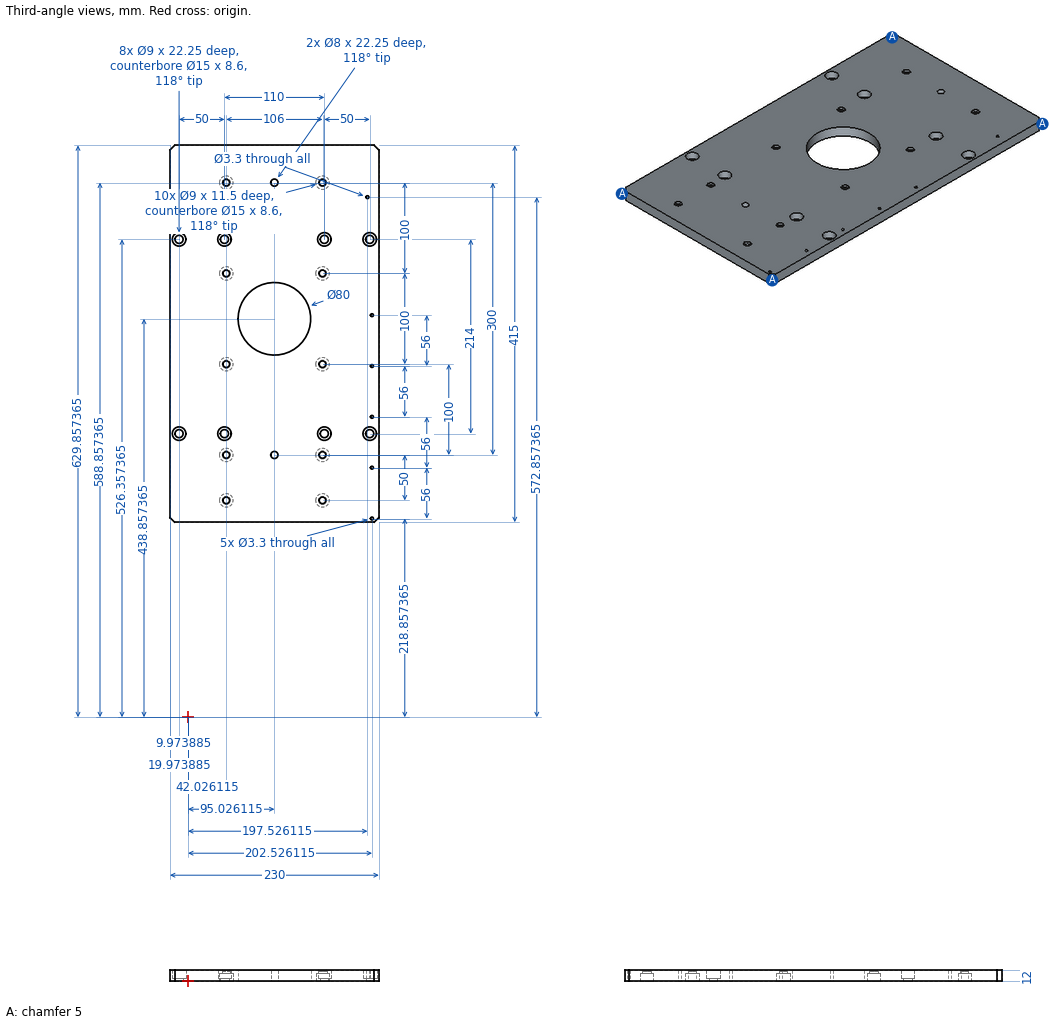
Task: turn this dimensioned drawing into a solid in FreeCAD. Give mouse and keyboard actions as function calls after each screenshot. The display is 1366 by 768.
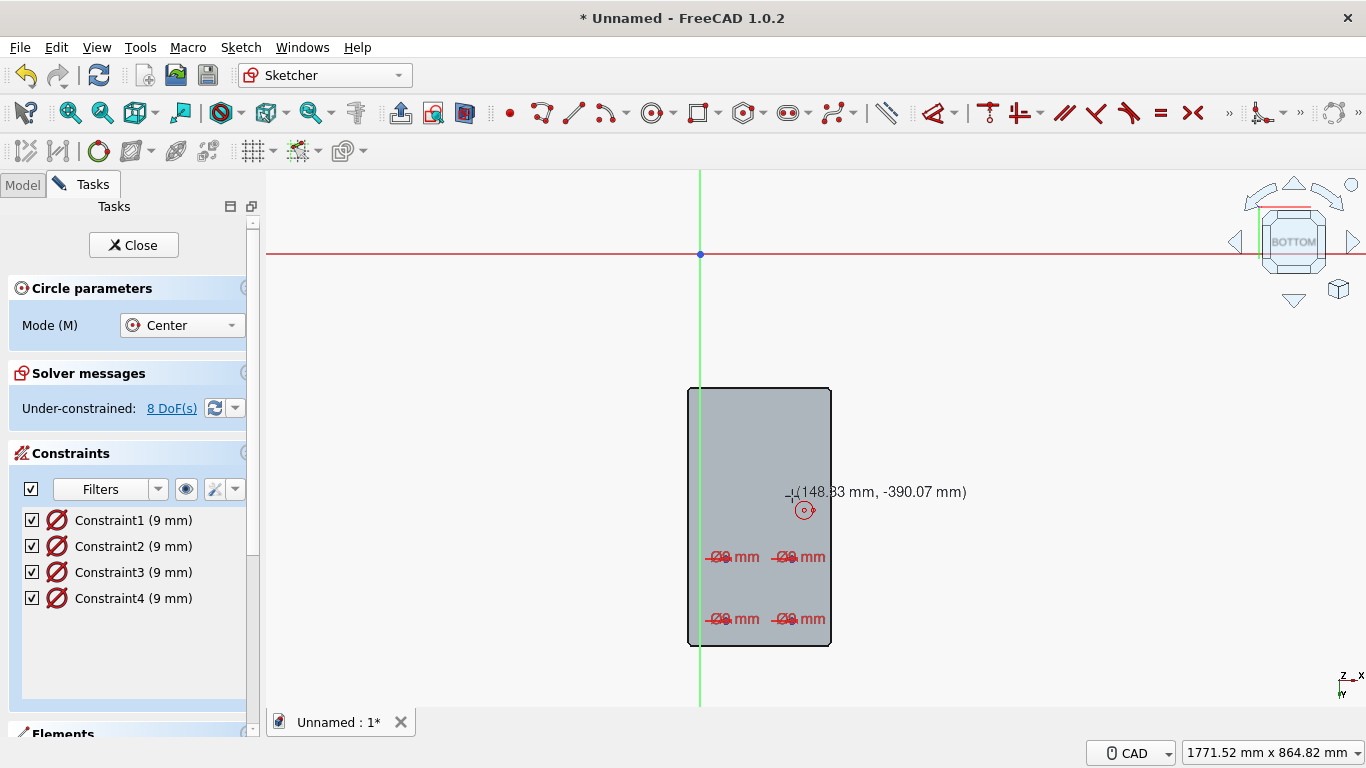
click(792, 496)
move(794, 494)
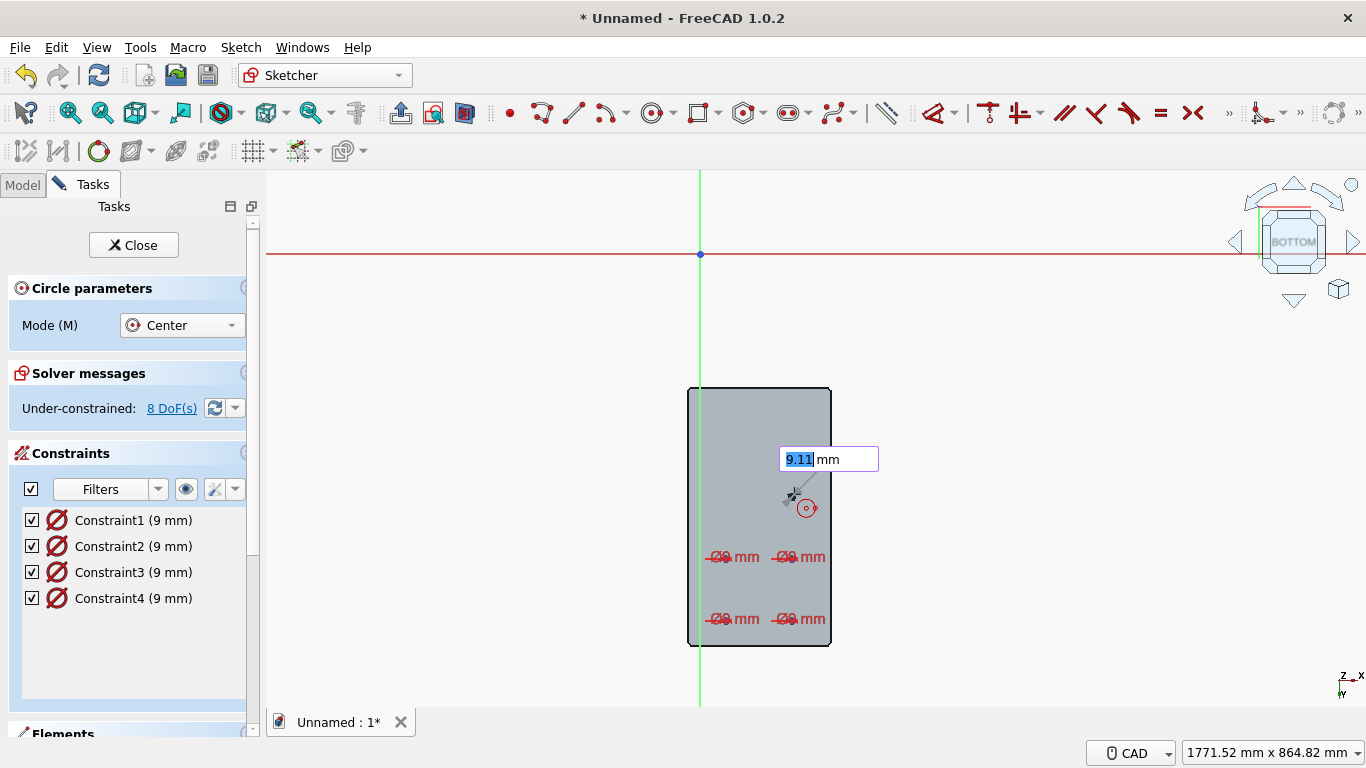
text(9)
key(Return)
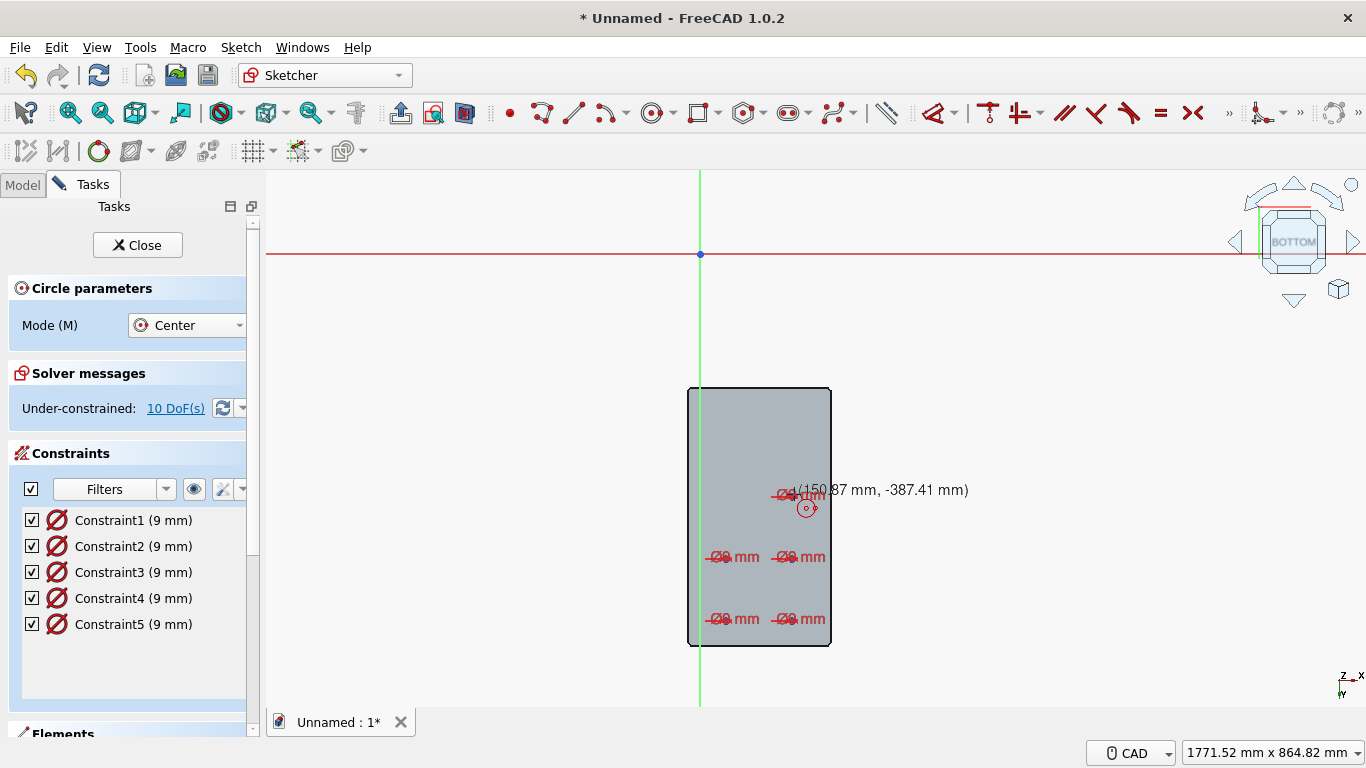
scroll(726, 496, up, 11)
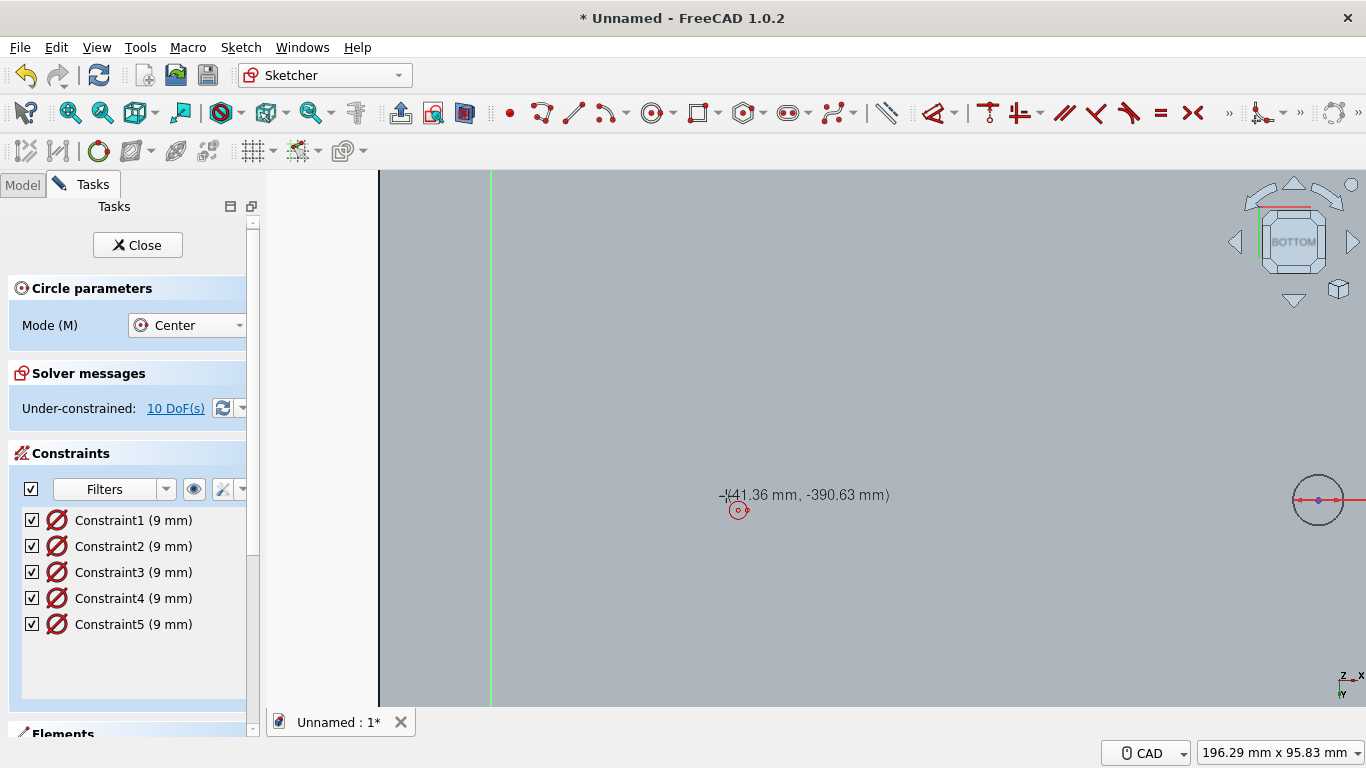
scroll(726, 496, down, 11)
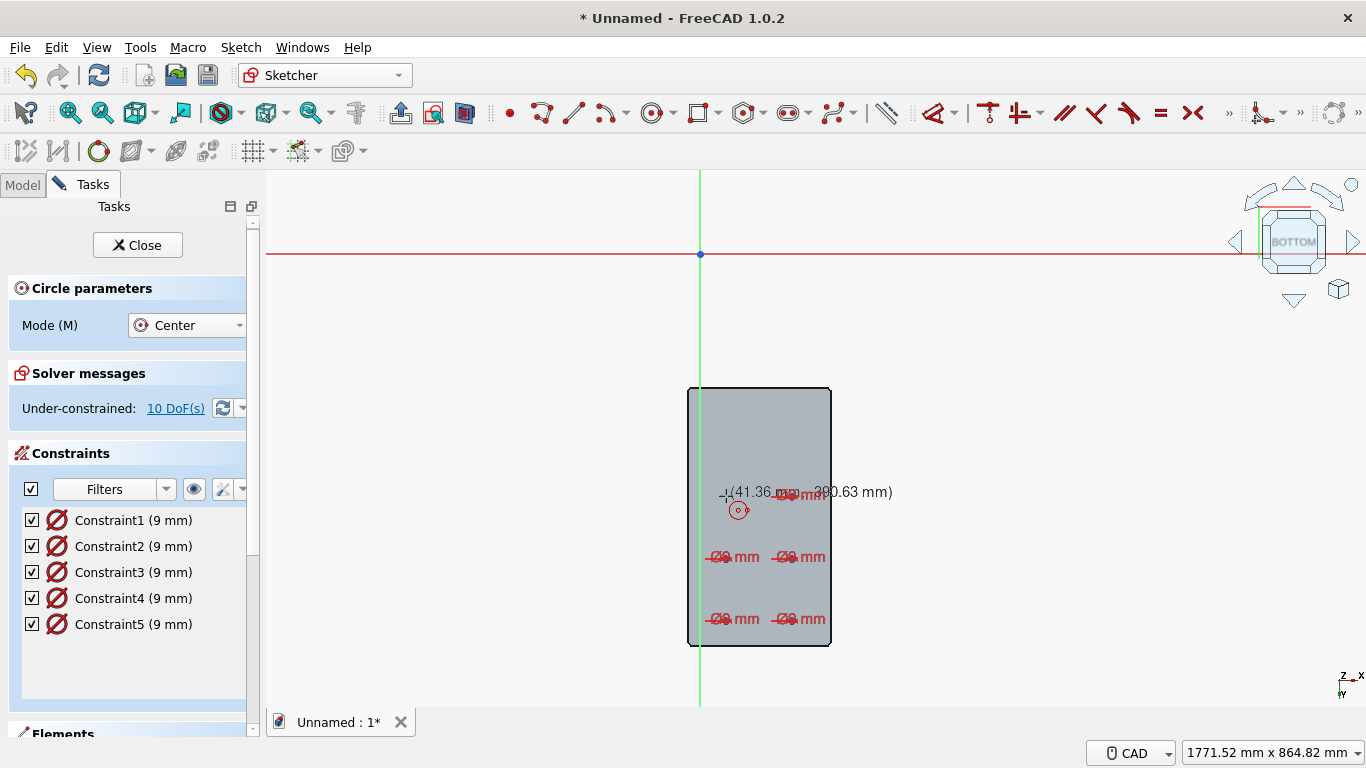
click(726, 496)
move(728, 494)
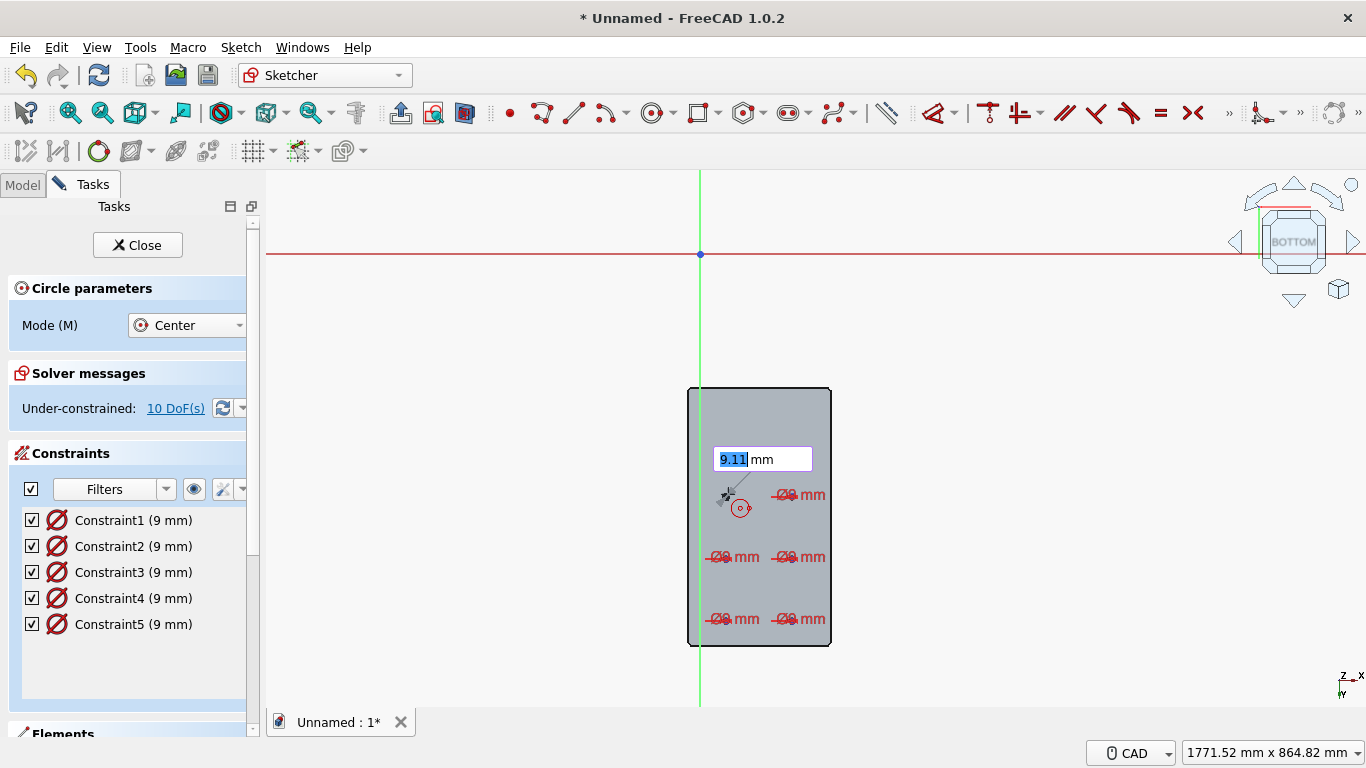
text(9)
key(Return)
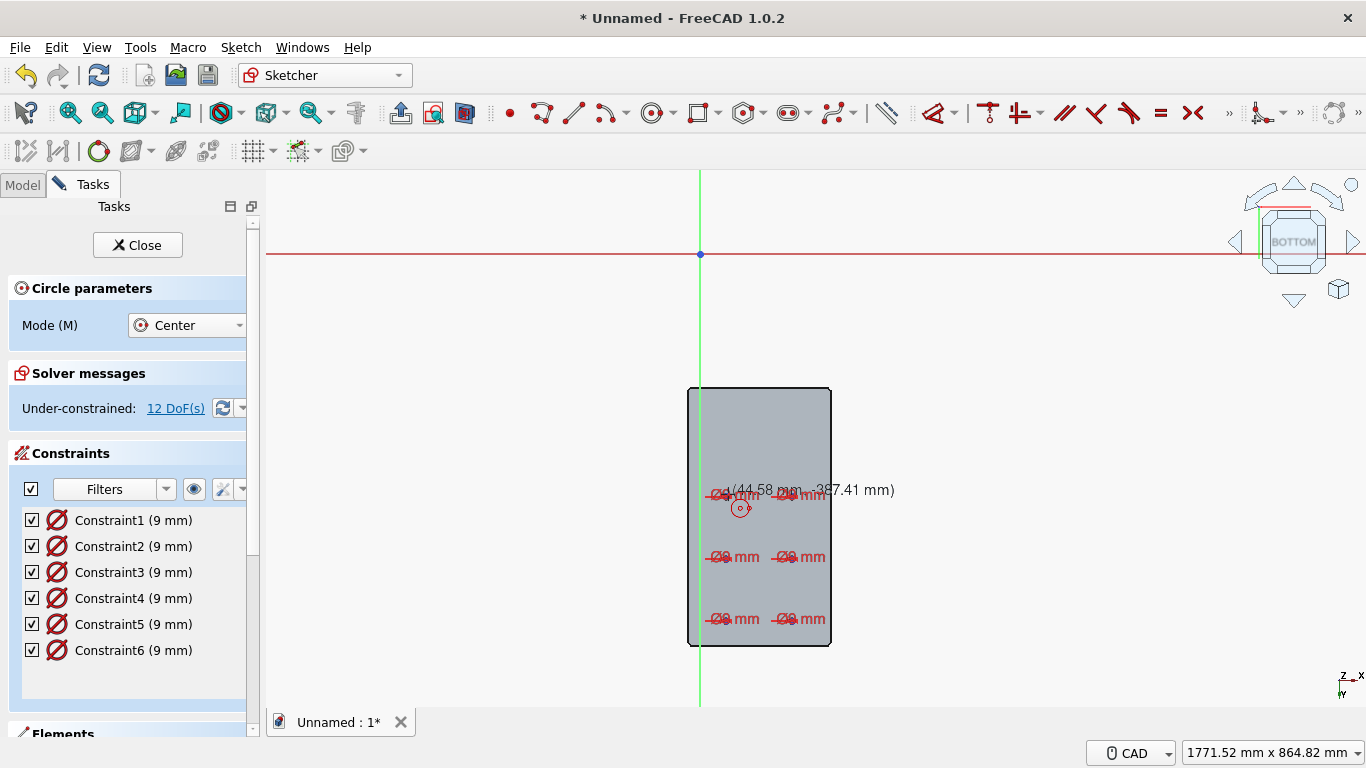
scroll(792, 434, up, 11)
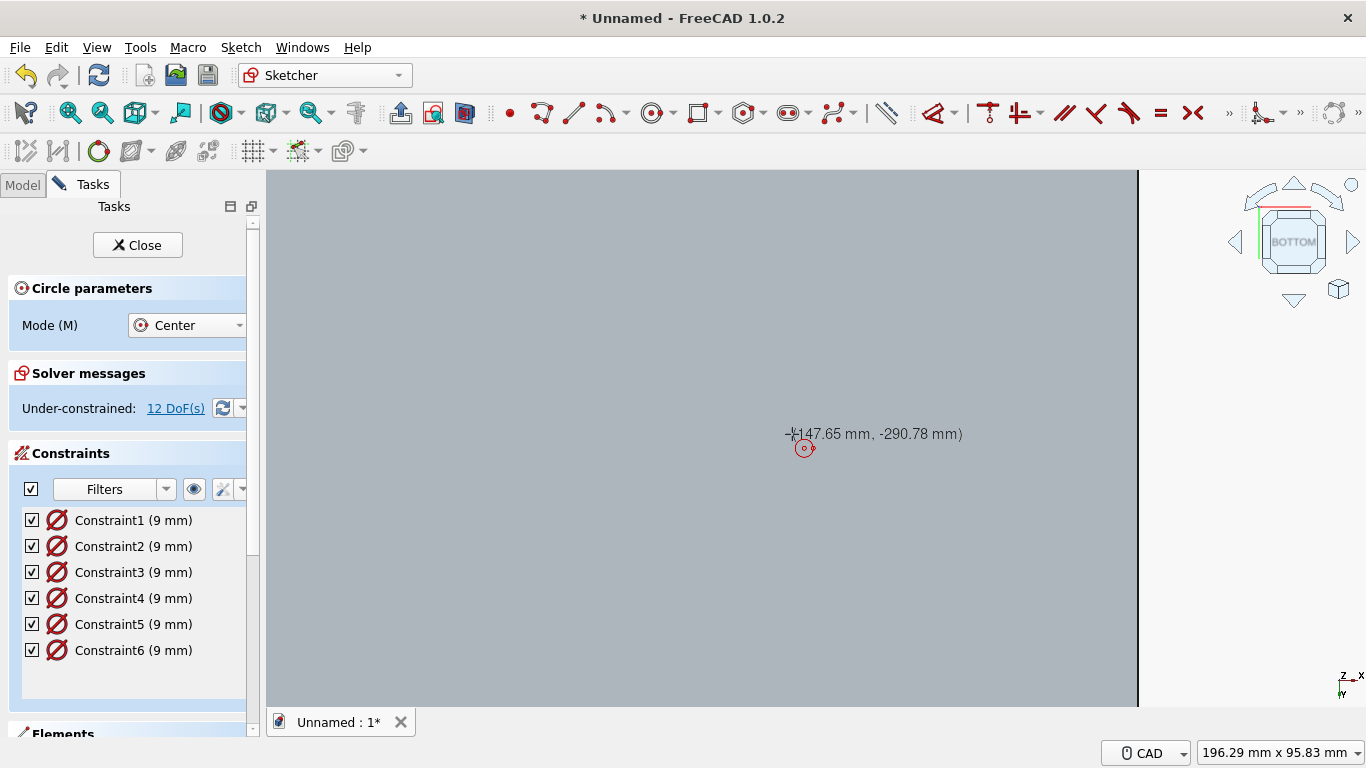
scroll(792, 434, down, 11)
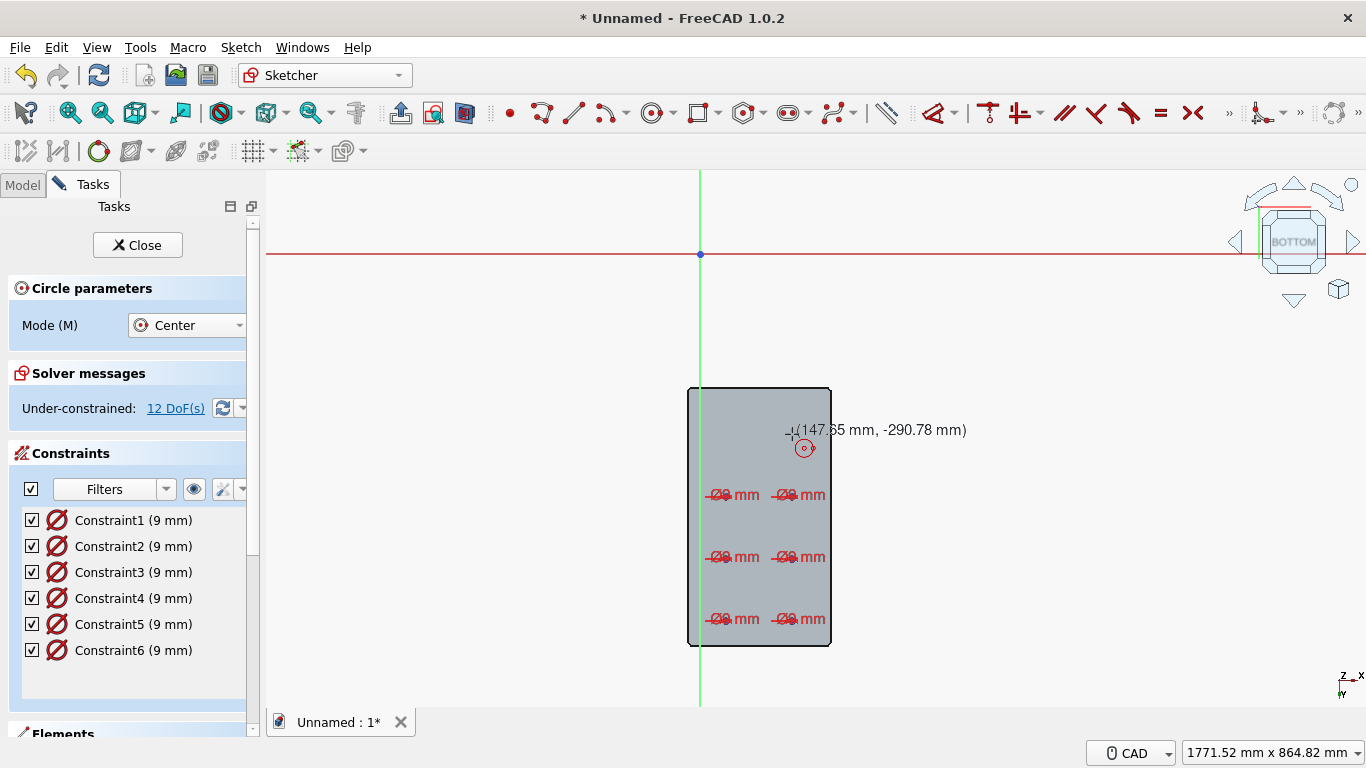
click(792, 434)
move(794, 432)